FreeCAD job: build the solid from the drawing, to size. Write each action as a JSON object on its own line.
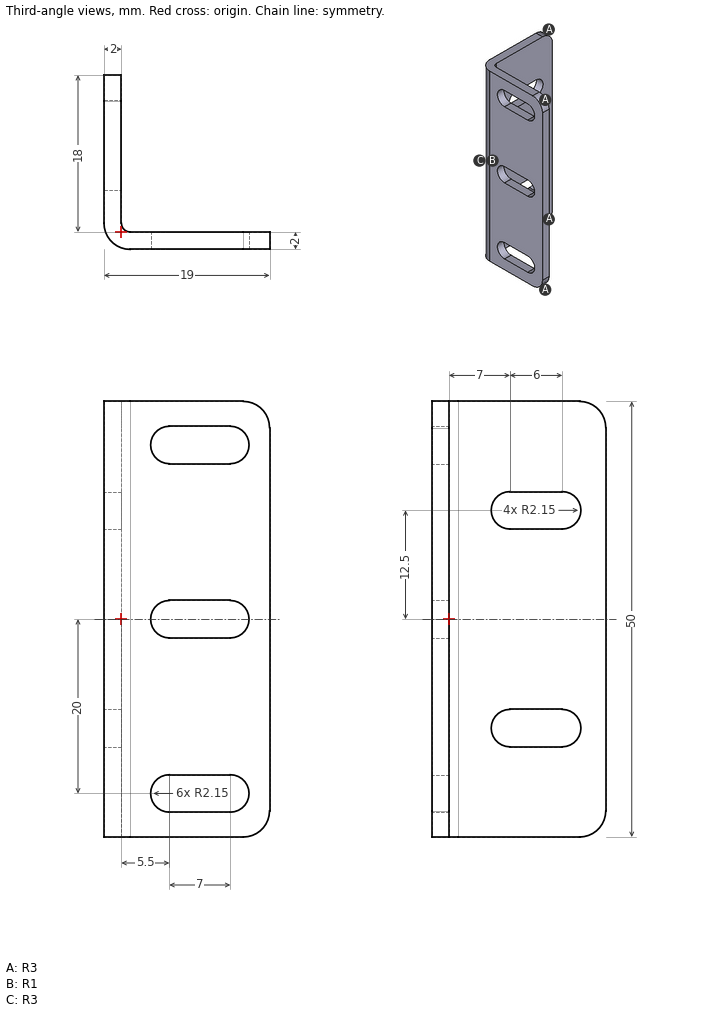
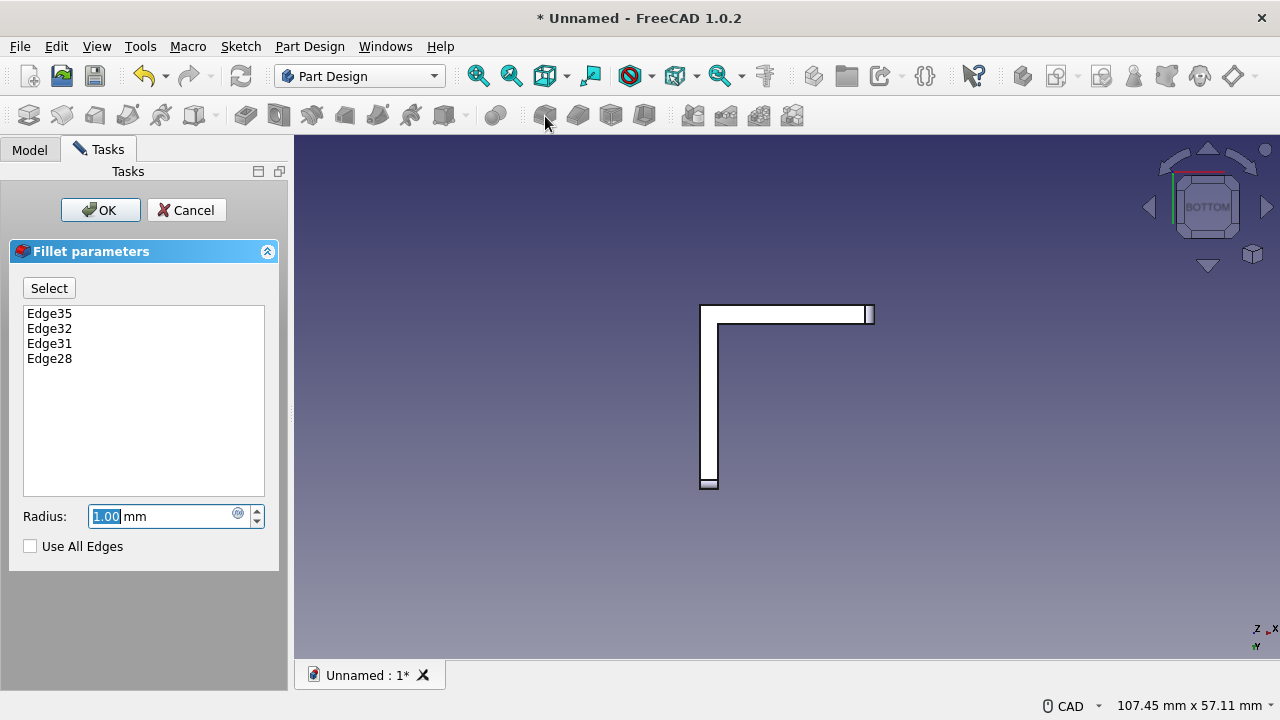
{"action": "type", "text": "3"}
{"action": "key", "text": "Tab"}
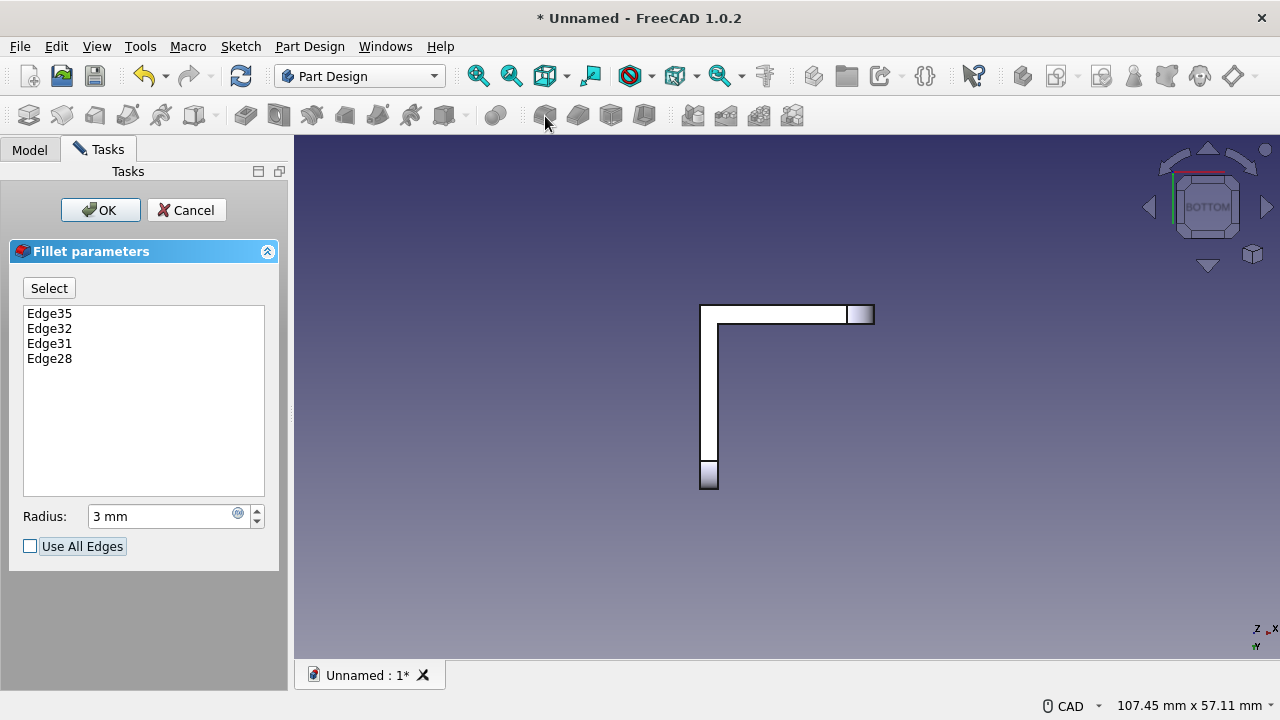
{"action": "left_click", "coordinate": [101, 210]}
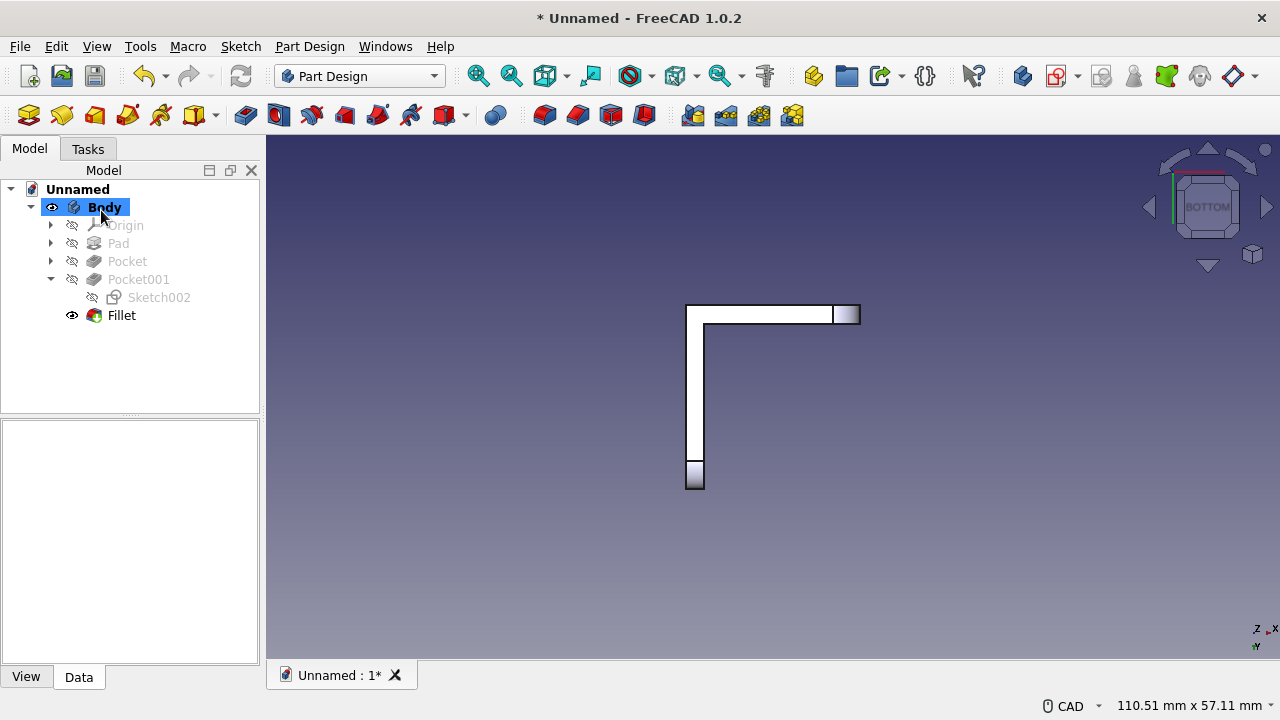
{"action": "left_click", "coordinate": [479, 76]}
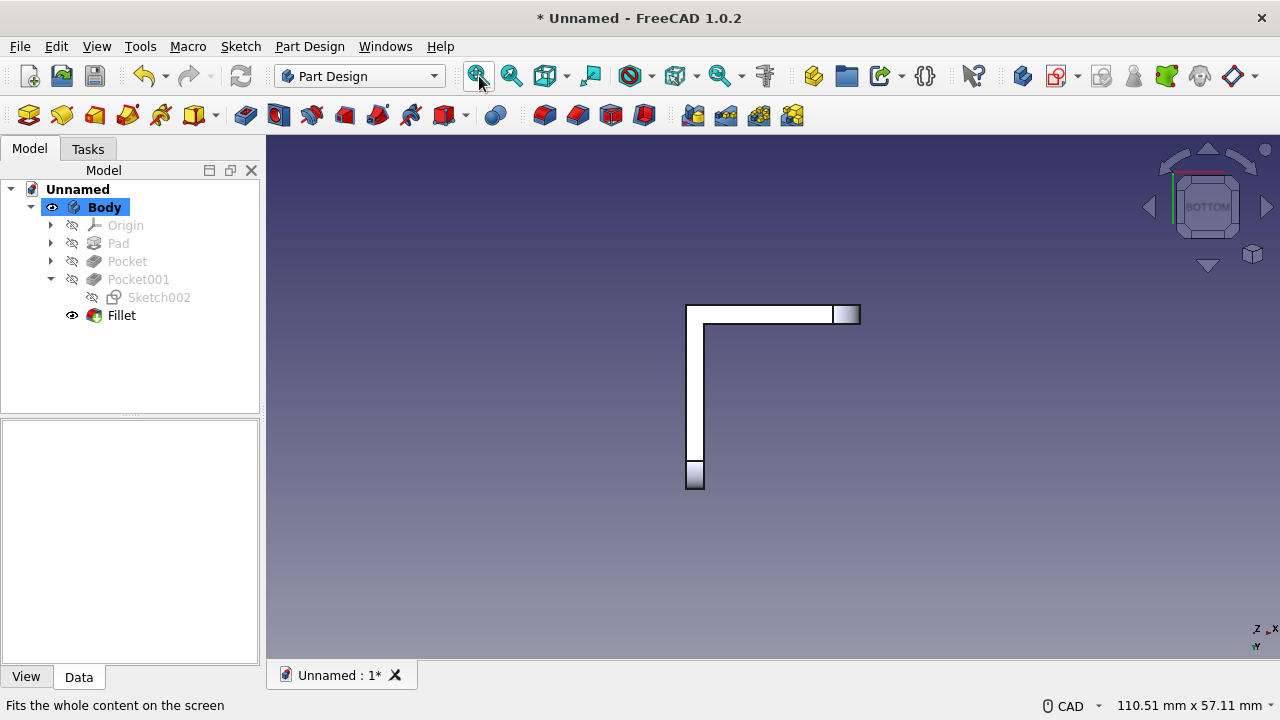
{"action": "key", "text": "0"}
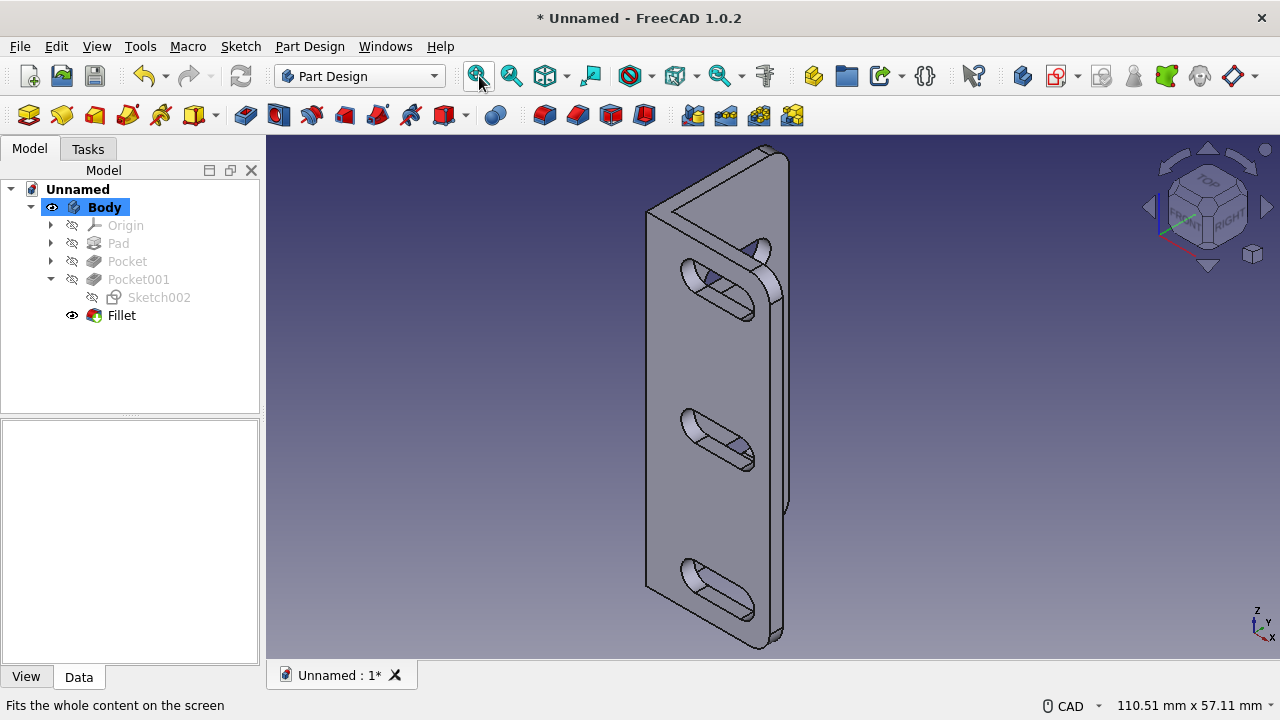
{"action": "key", "text": "2"}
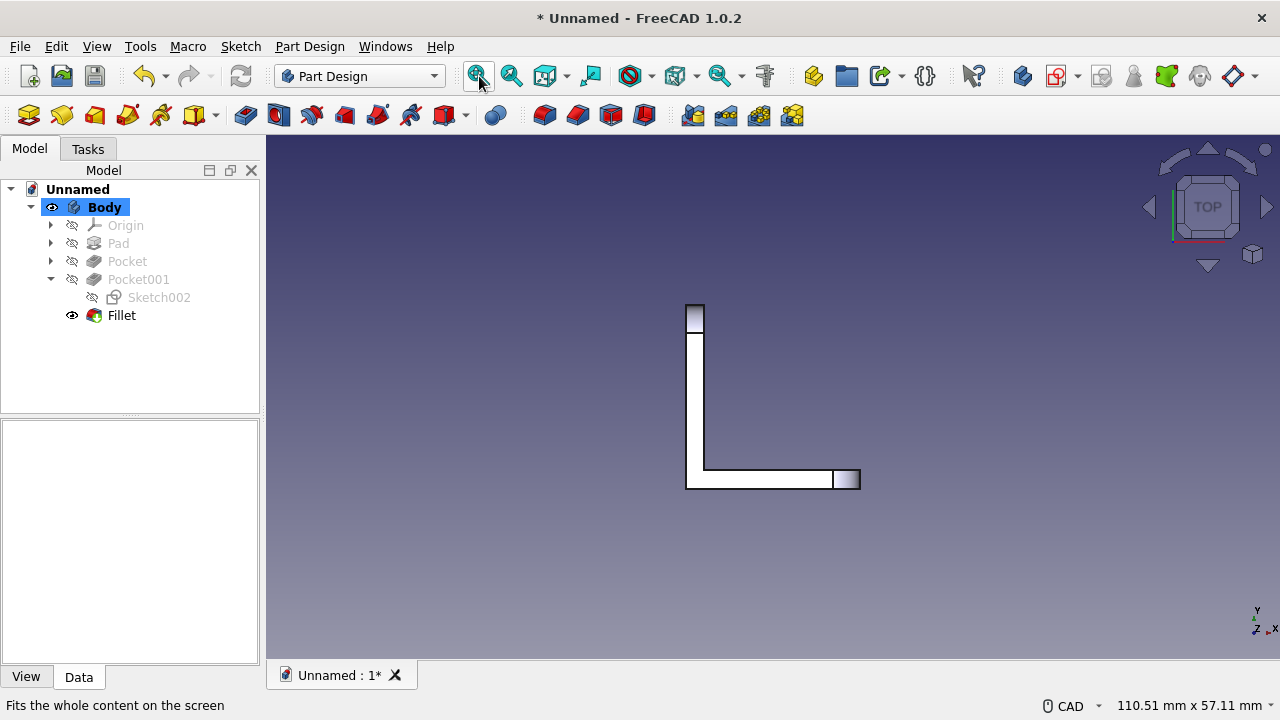
{"action": "left_click", "coordinate": [479, 76]}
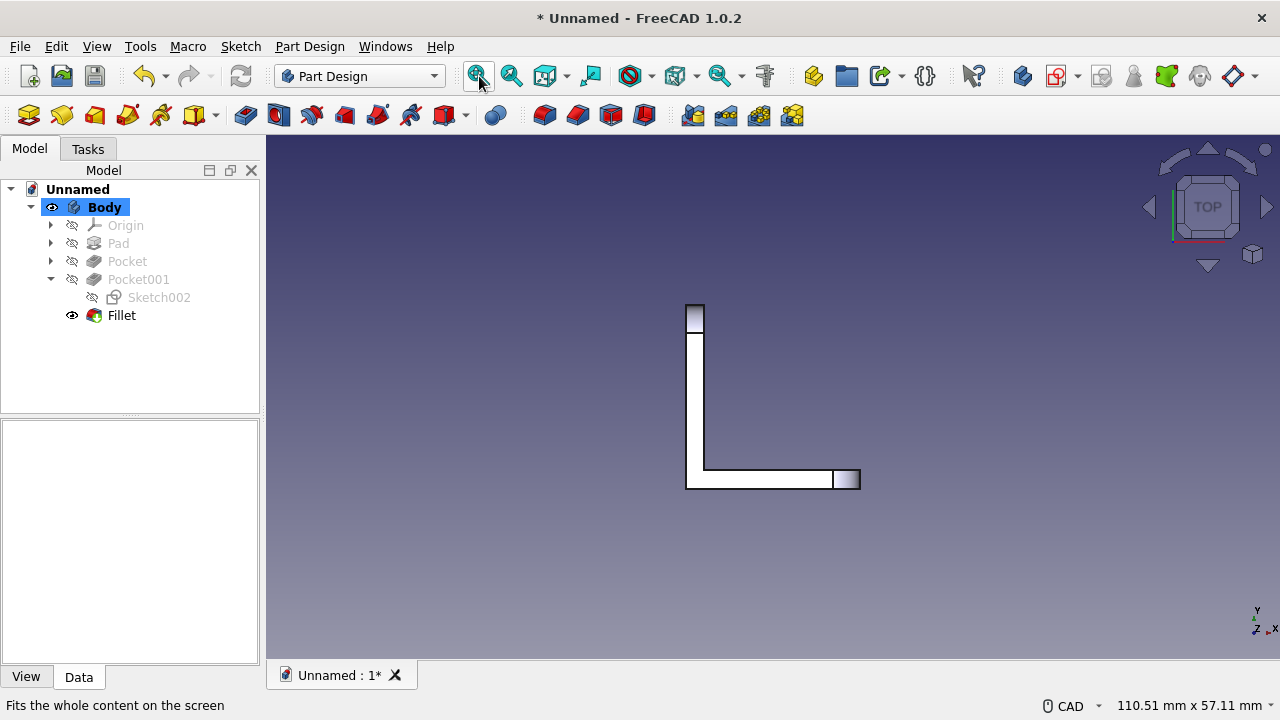
{"action": "key", "text": "1"}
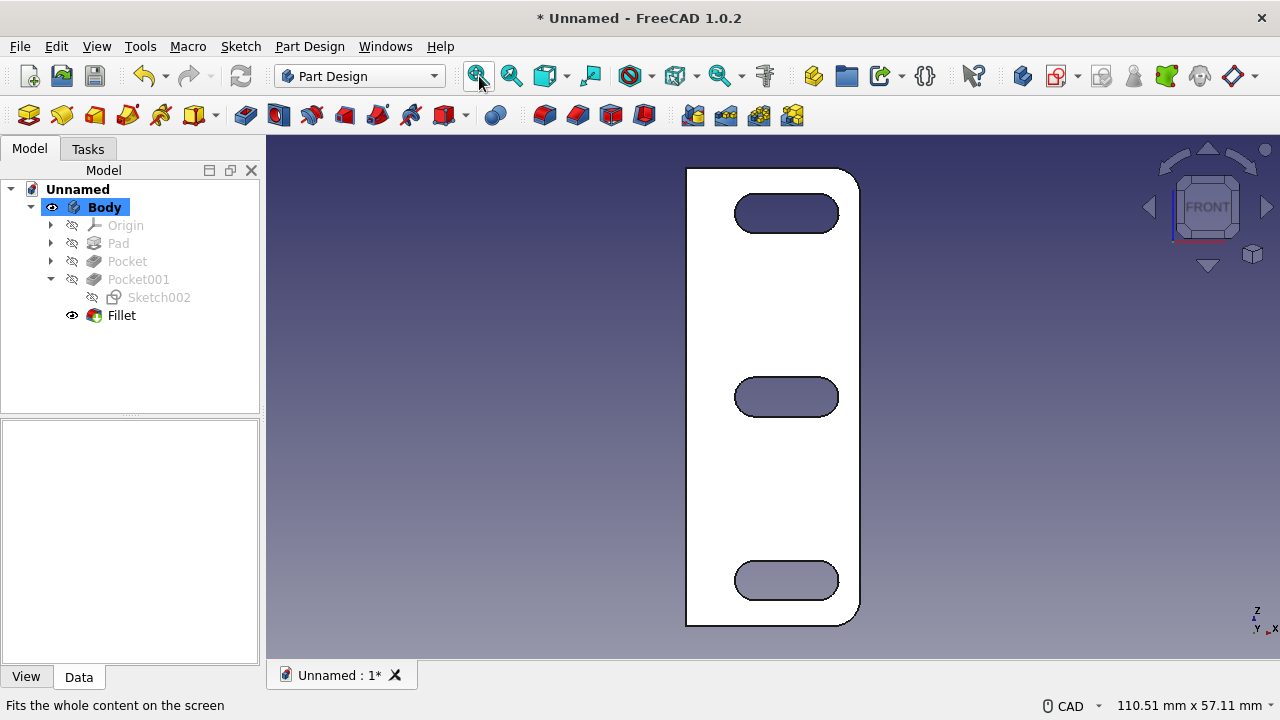
{"action": "key", "text": "3"}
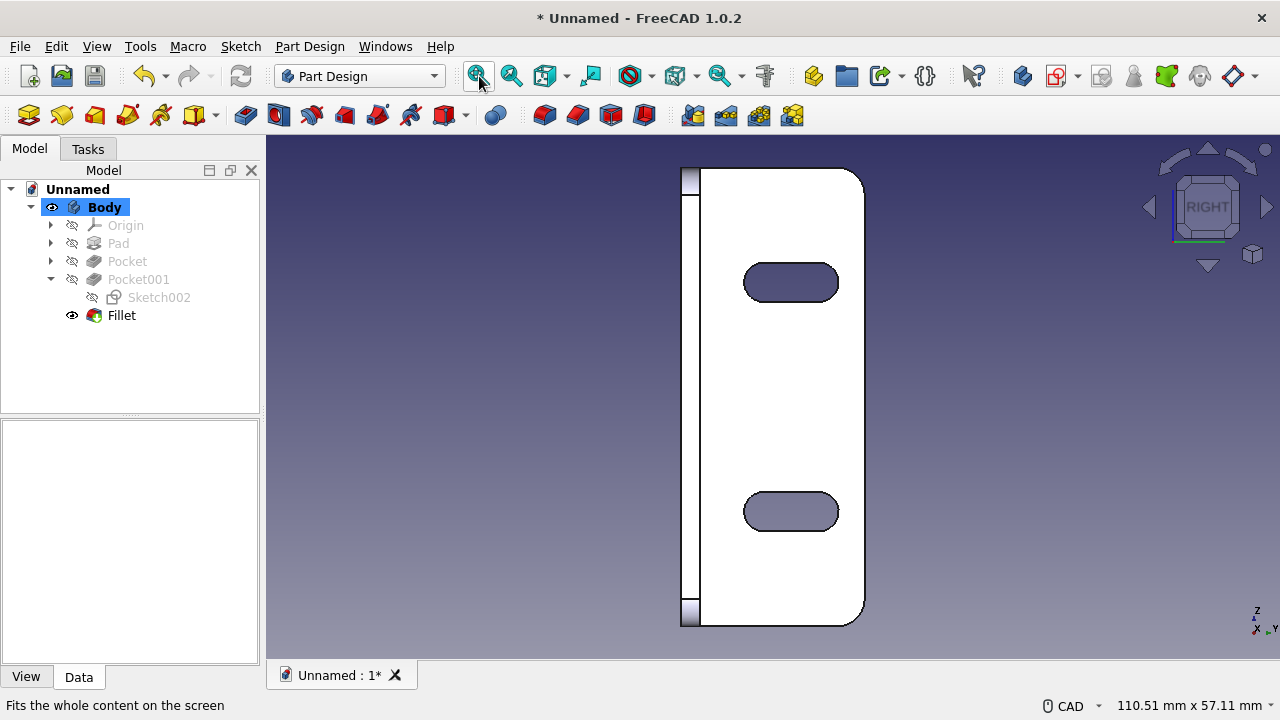
{"action": "key", "text": "5"}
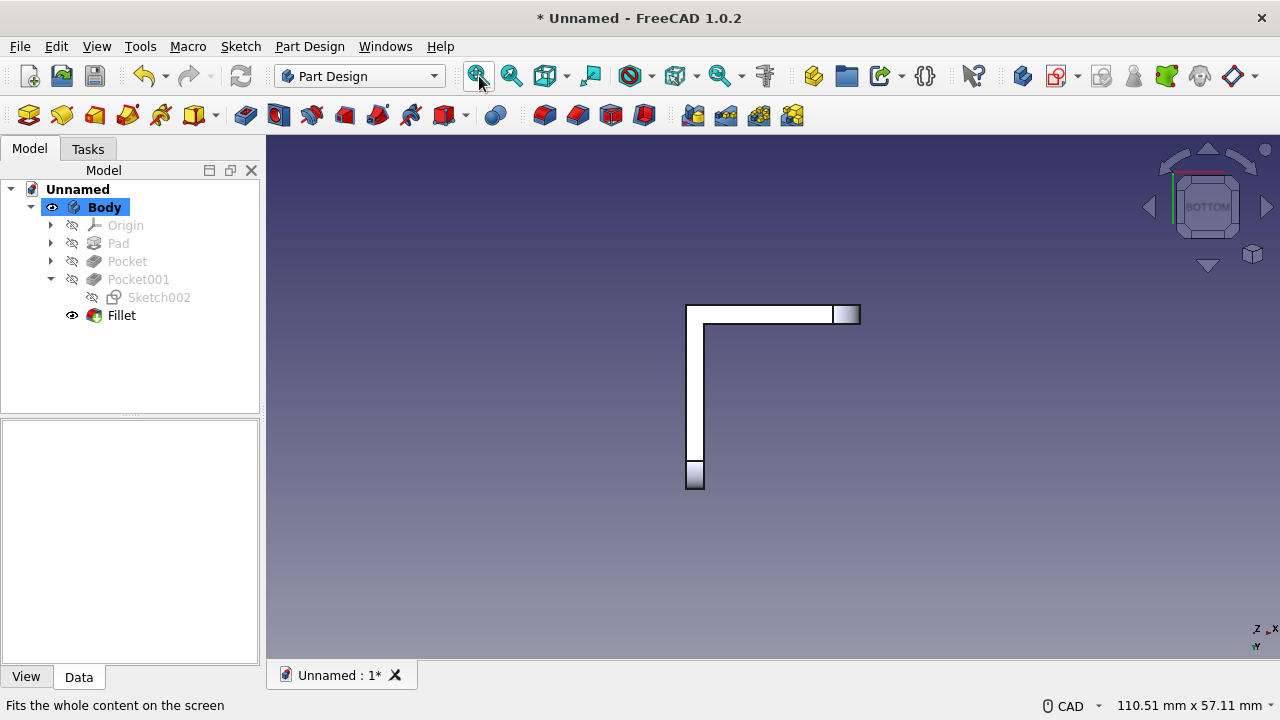
{"action": "left_click", "coordinate": [479, 76]}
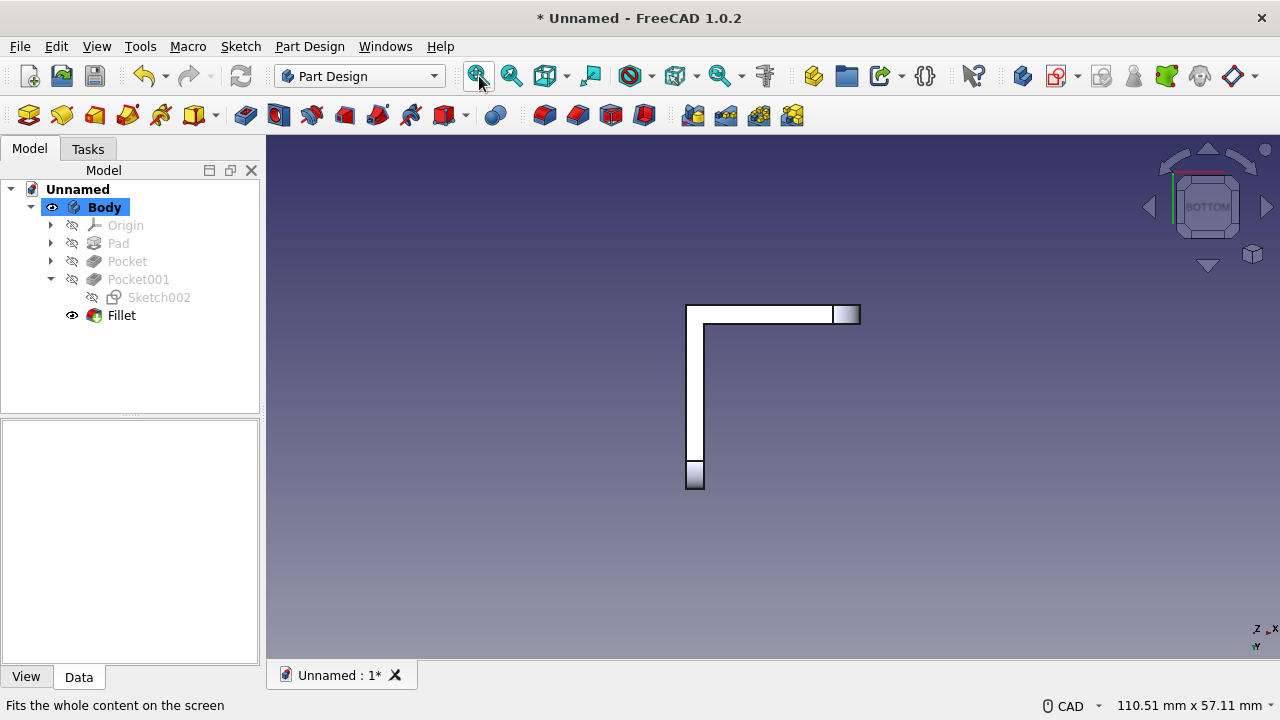
{"action": "key", "text": "4"}